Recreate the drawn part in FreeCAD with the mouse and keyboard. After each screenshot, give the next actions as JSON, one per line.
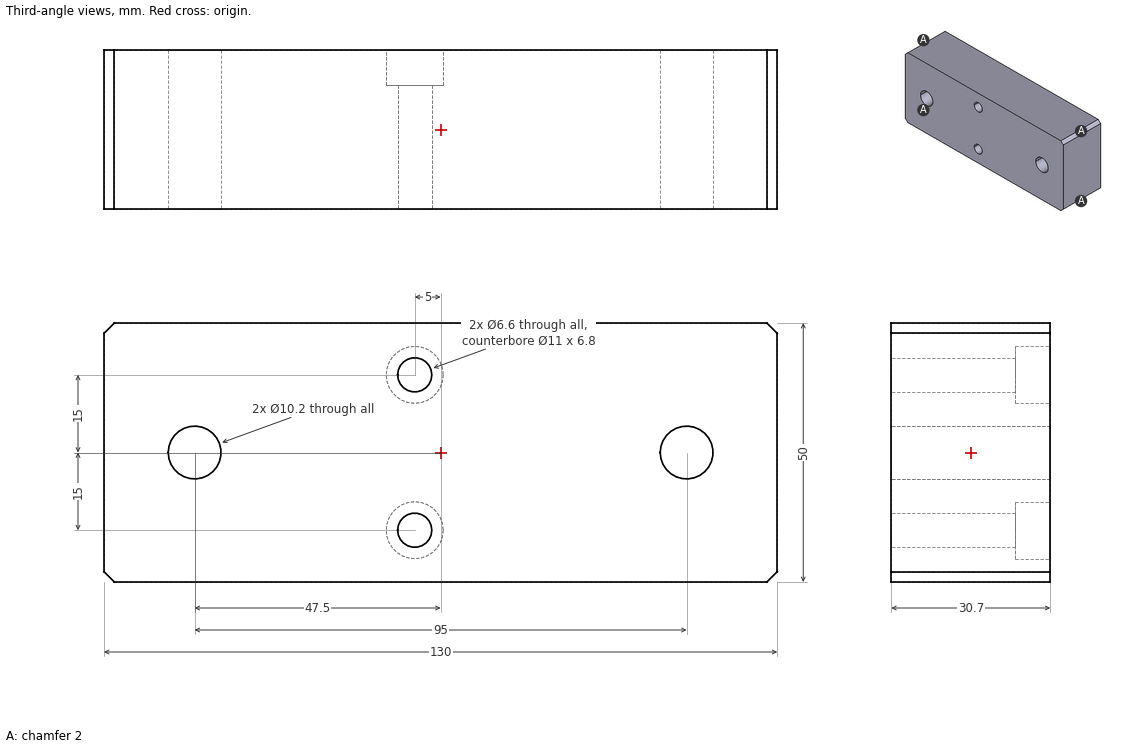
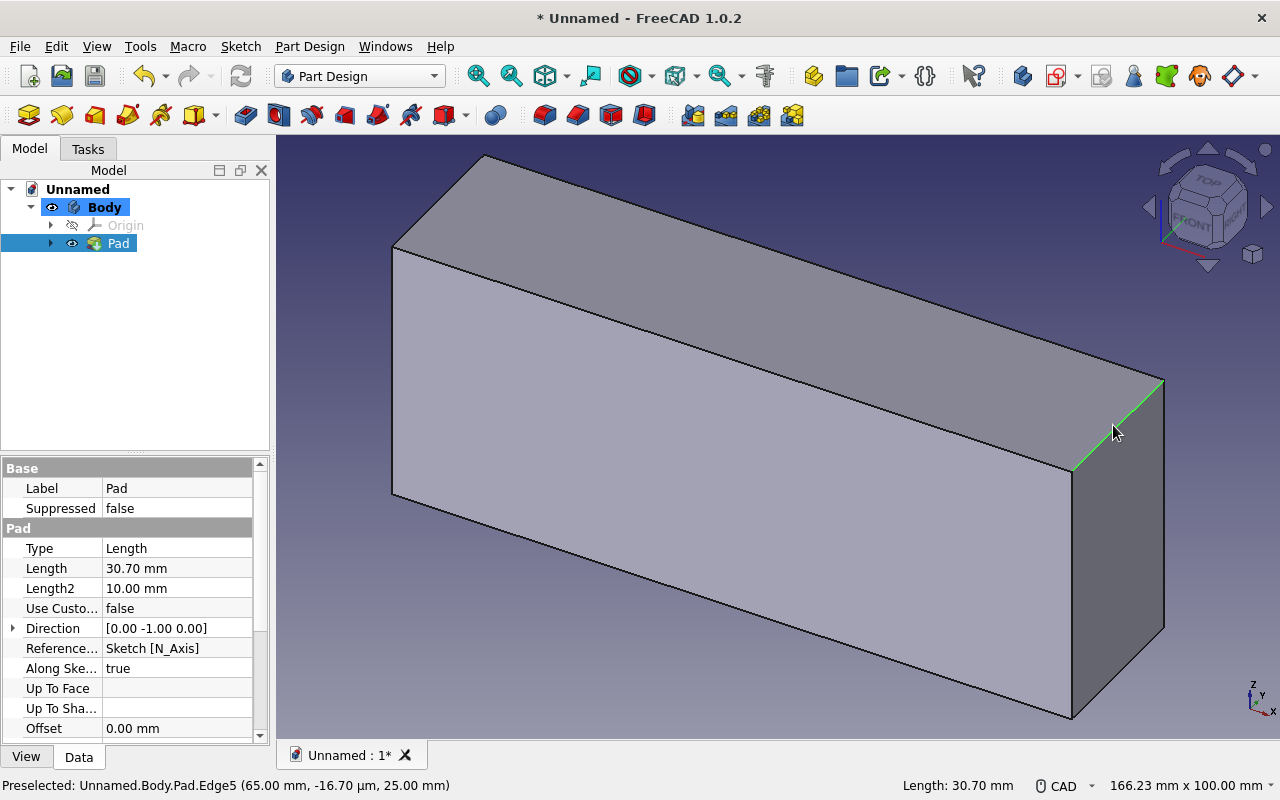
{"action": "key", "text": "0"}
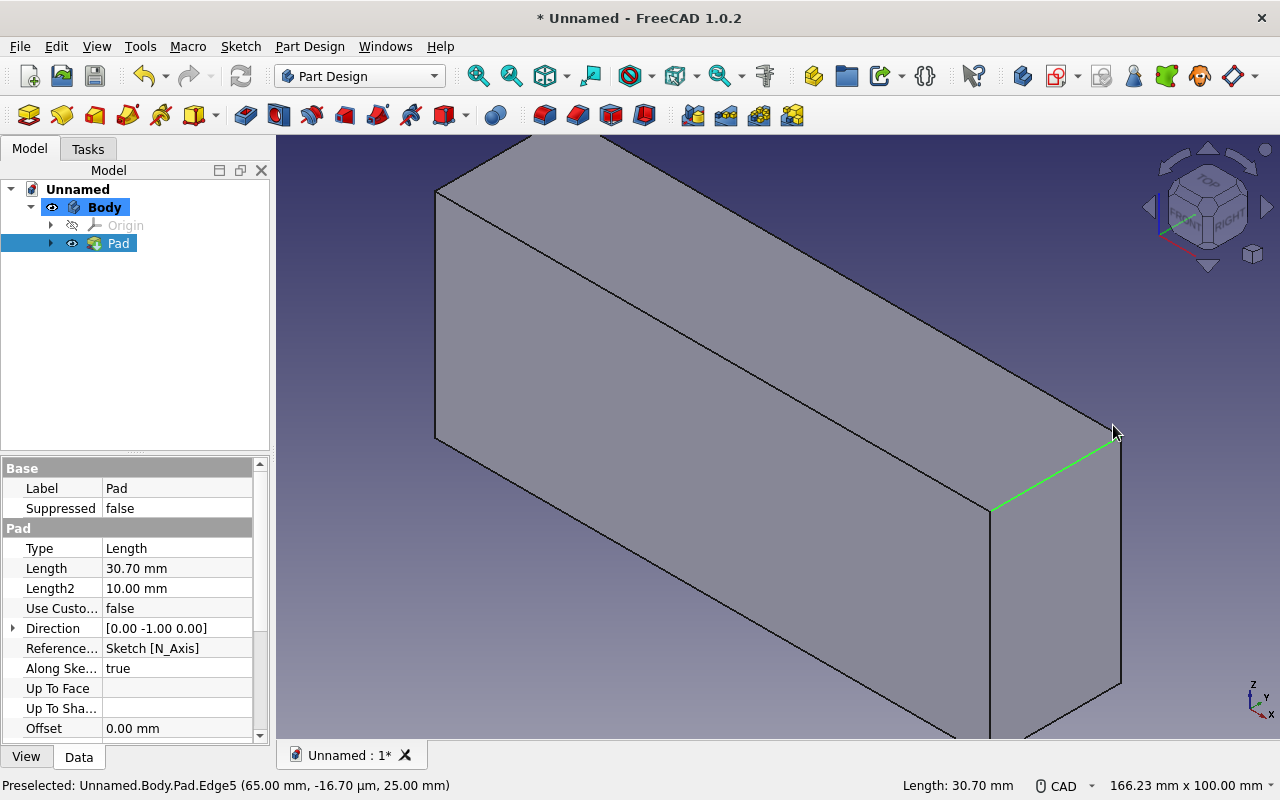
{"action": "left_click", "coordinate": [479, 76]}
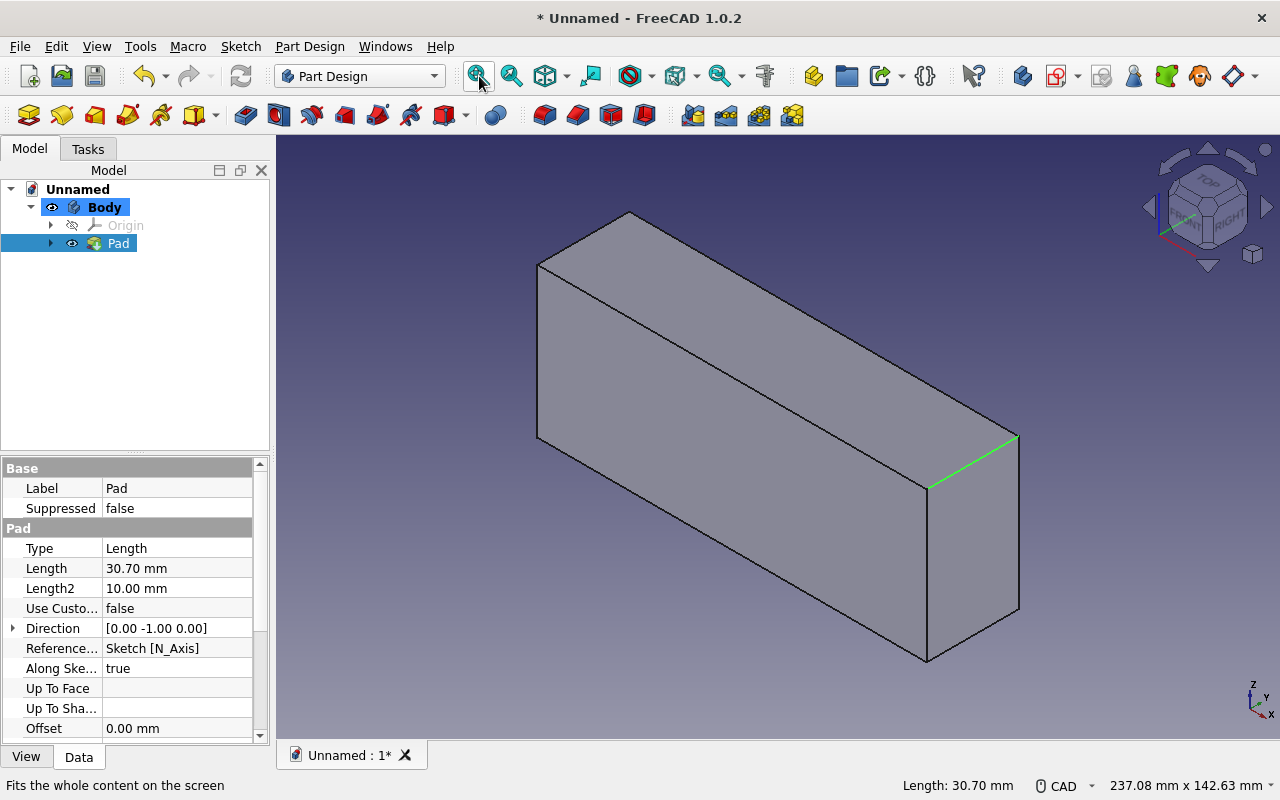
{"action": "key", "text": "2"}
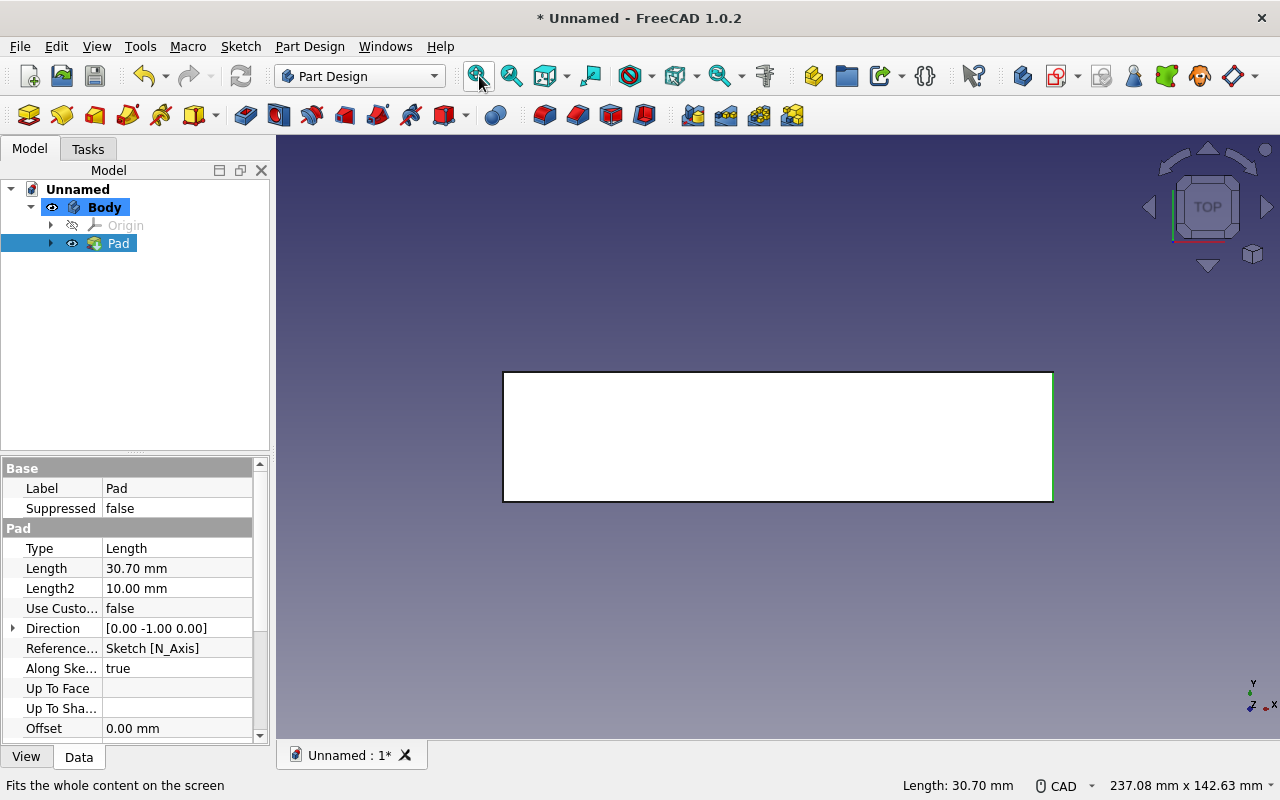
{"action": "left_click", "coordinate": [503, 436], "text": "ctrl"}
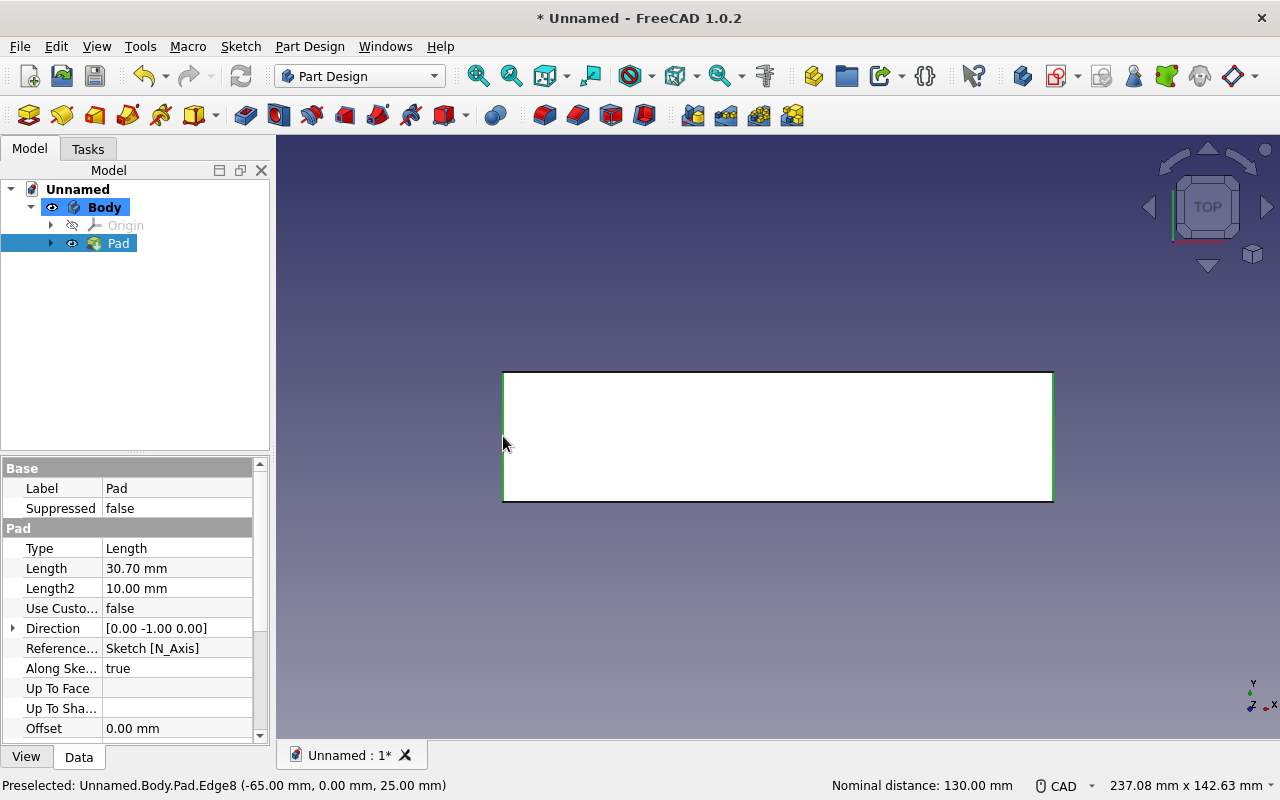
{"action": "key", "text": "1"}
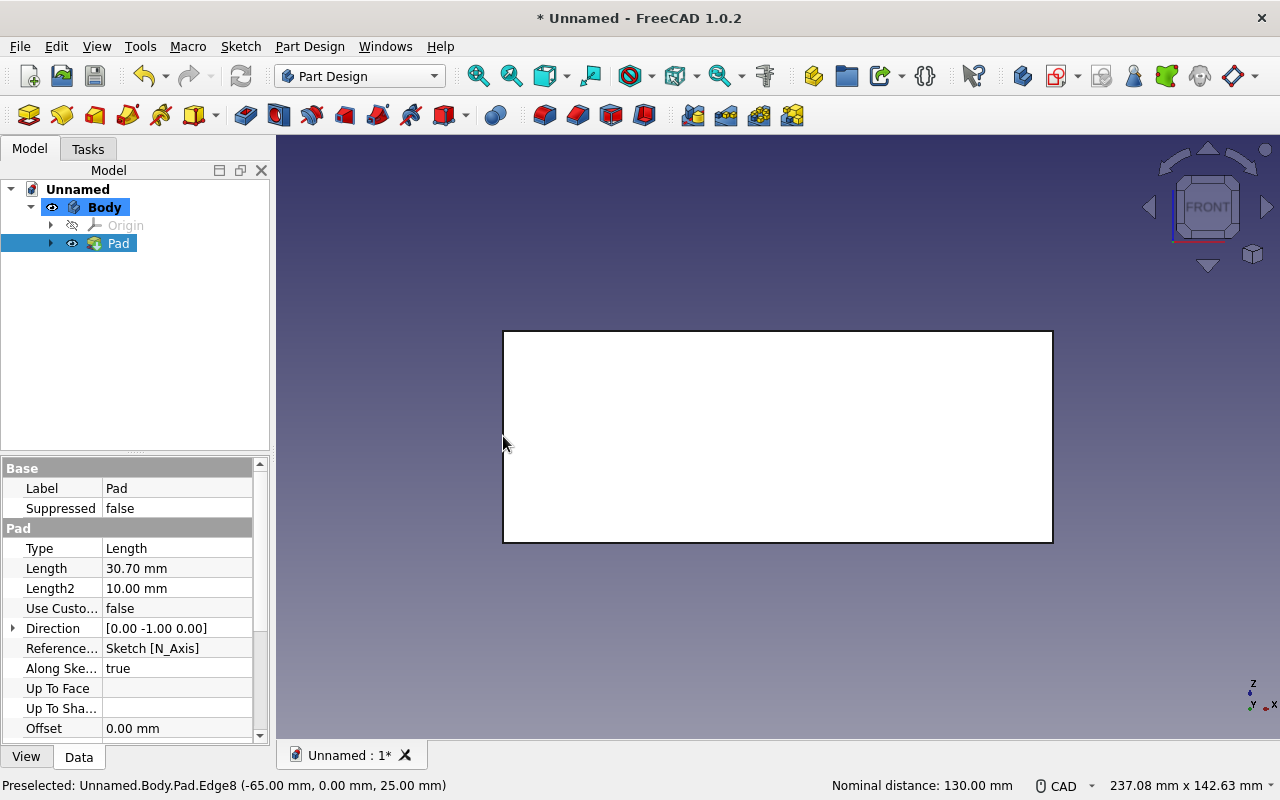
{"action": "key", "text": "3"}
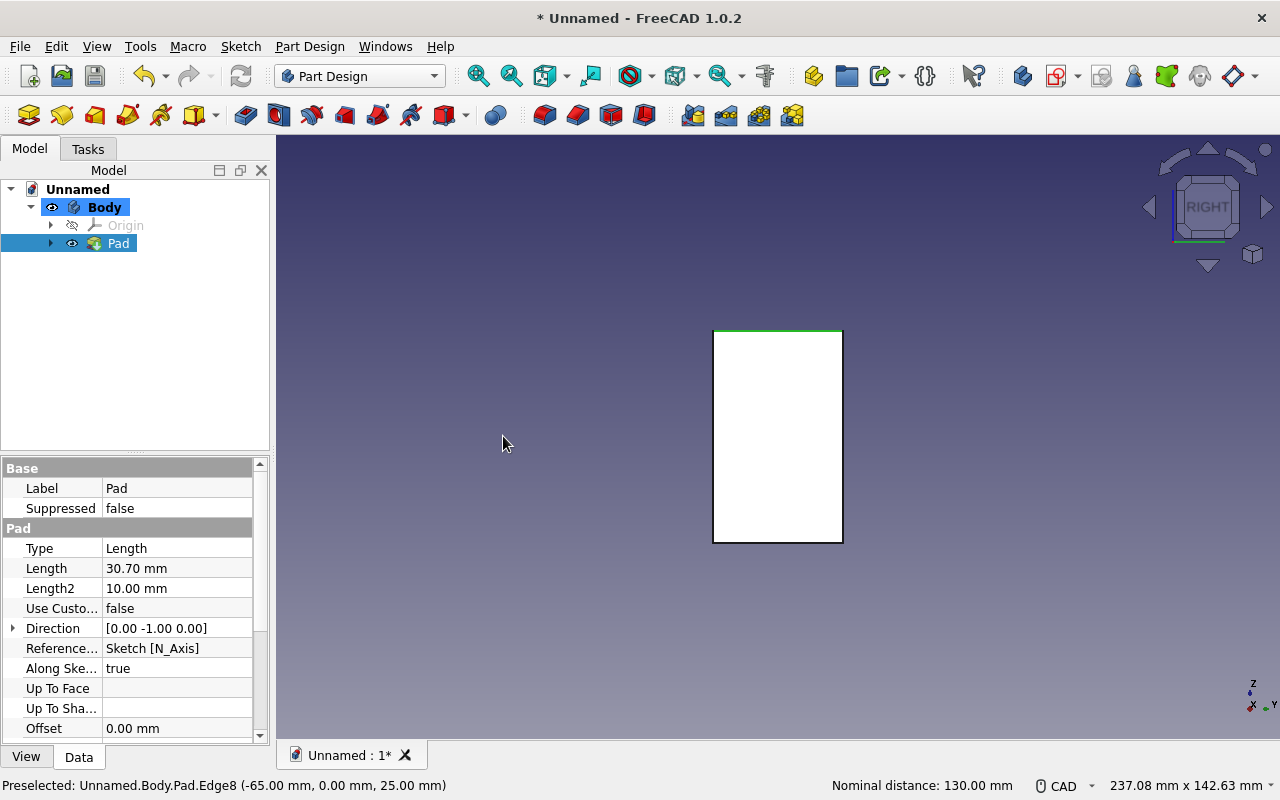
{"action": "left_click", "coordinate": [479, 76]}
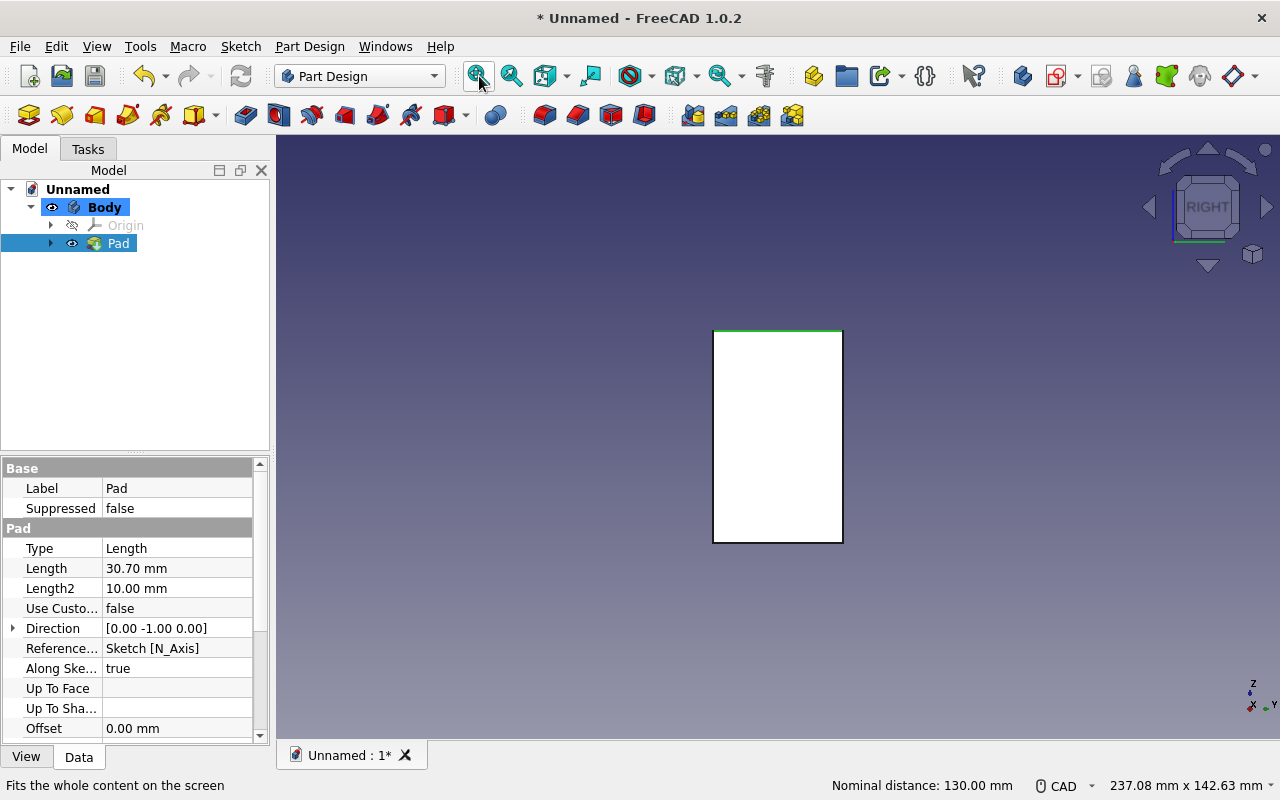
{"action": "left_click", "coordinate": [778, 542], "text": "ctrl"}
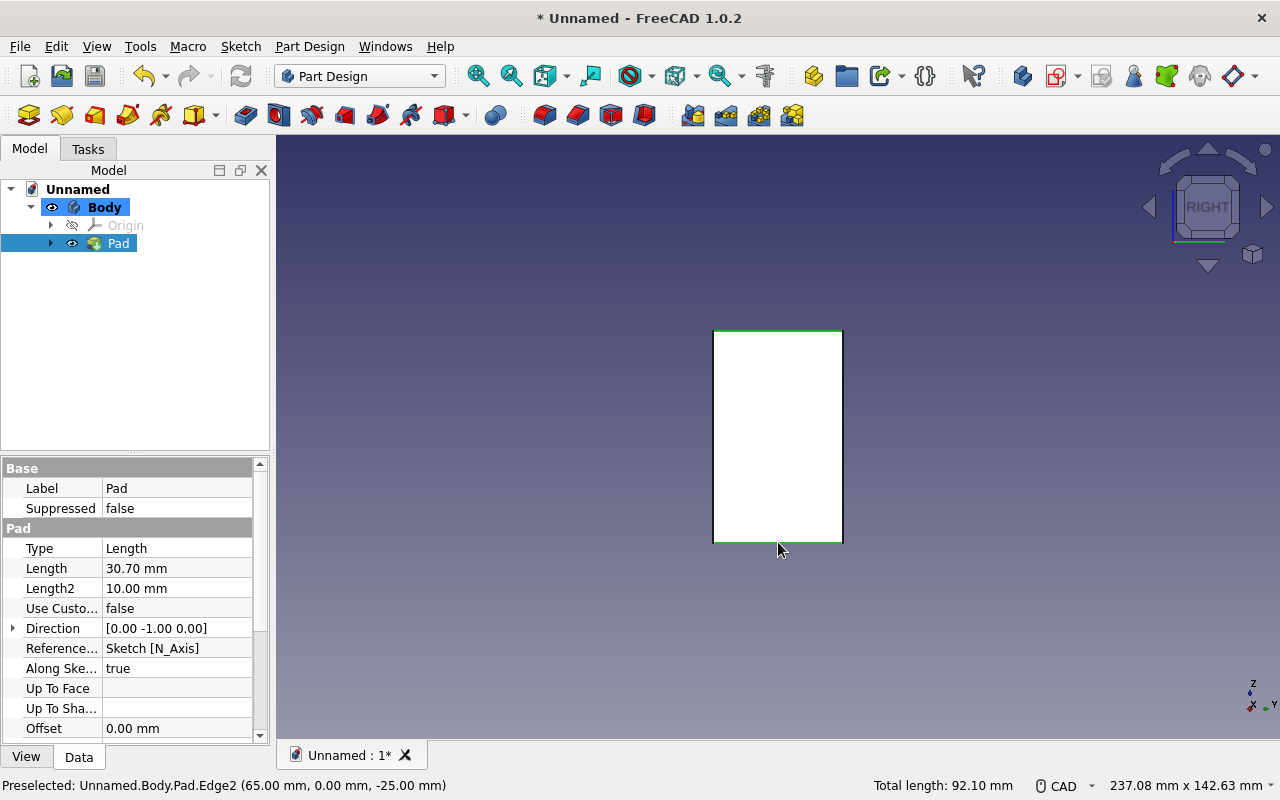
{"action": "key", "text": "5"}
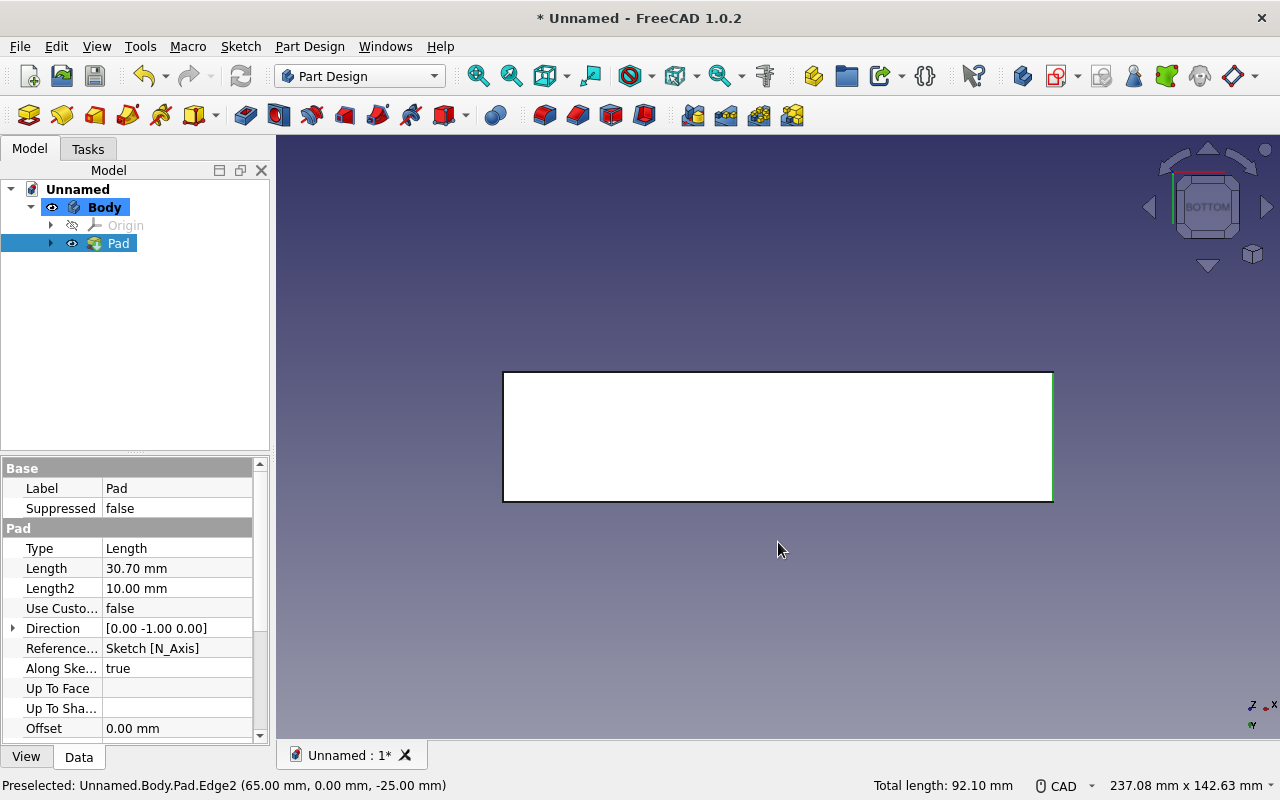
{"action": "left_click", "coordinate": [503, 436], "text": "ctrl"}